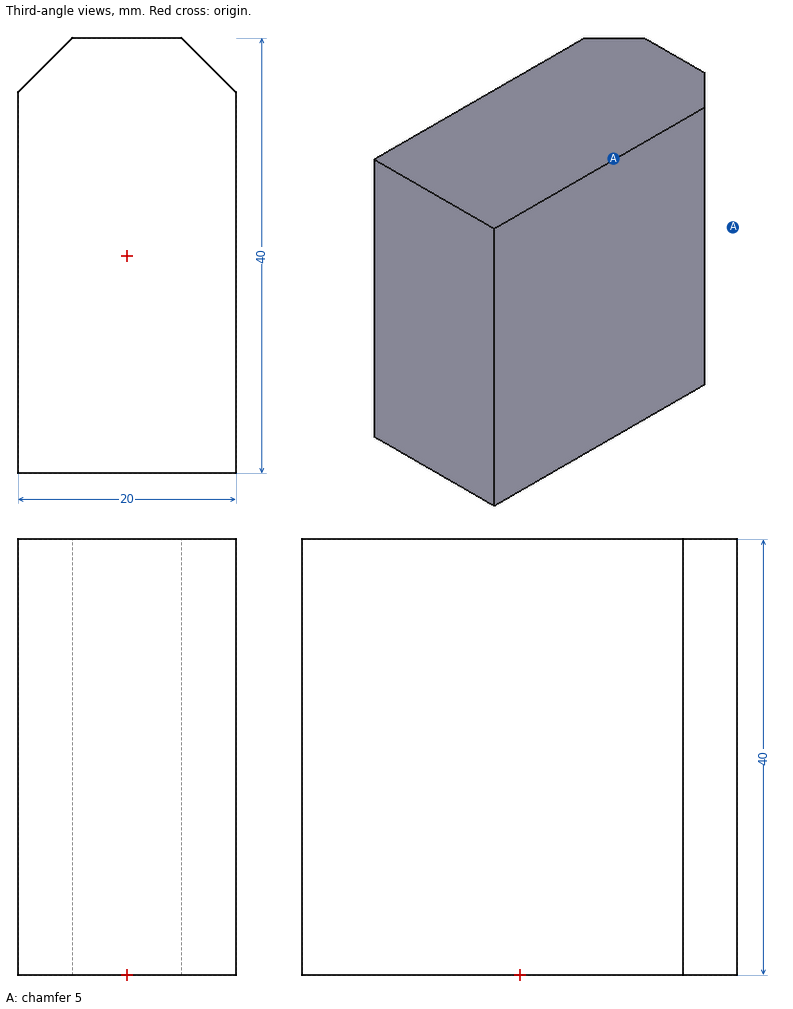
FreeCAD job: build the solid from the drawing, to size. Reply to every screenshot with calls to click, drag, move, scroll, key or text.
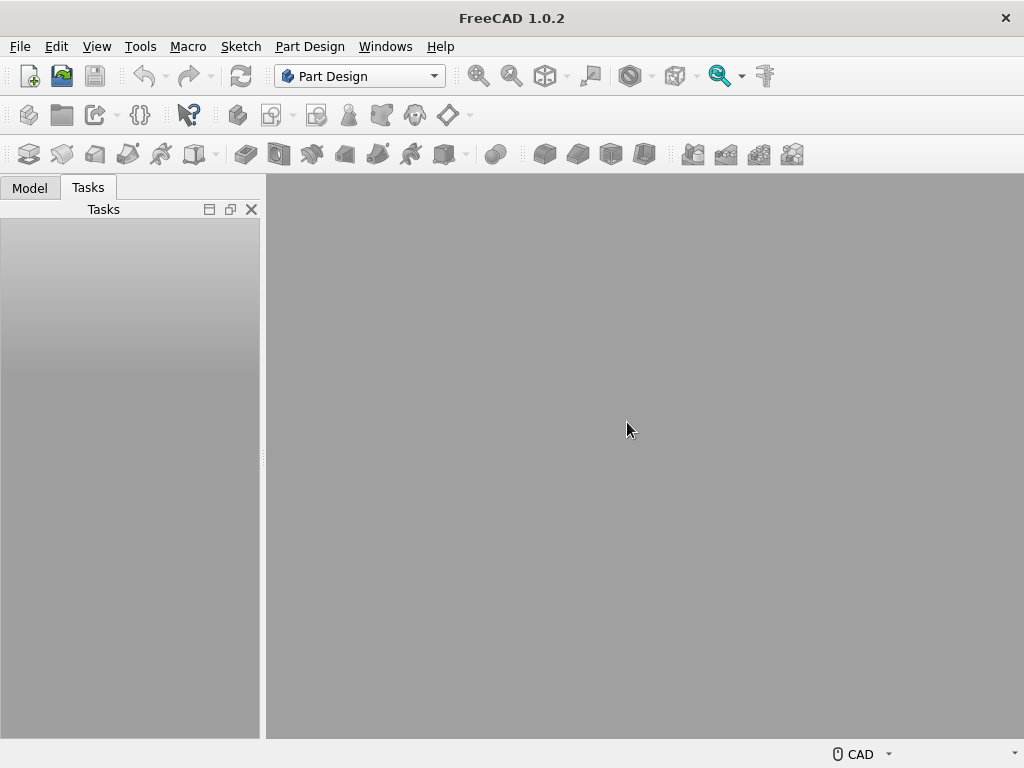
click(29, 76)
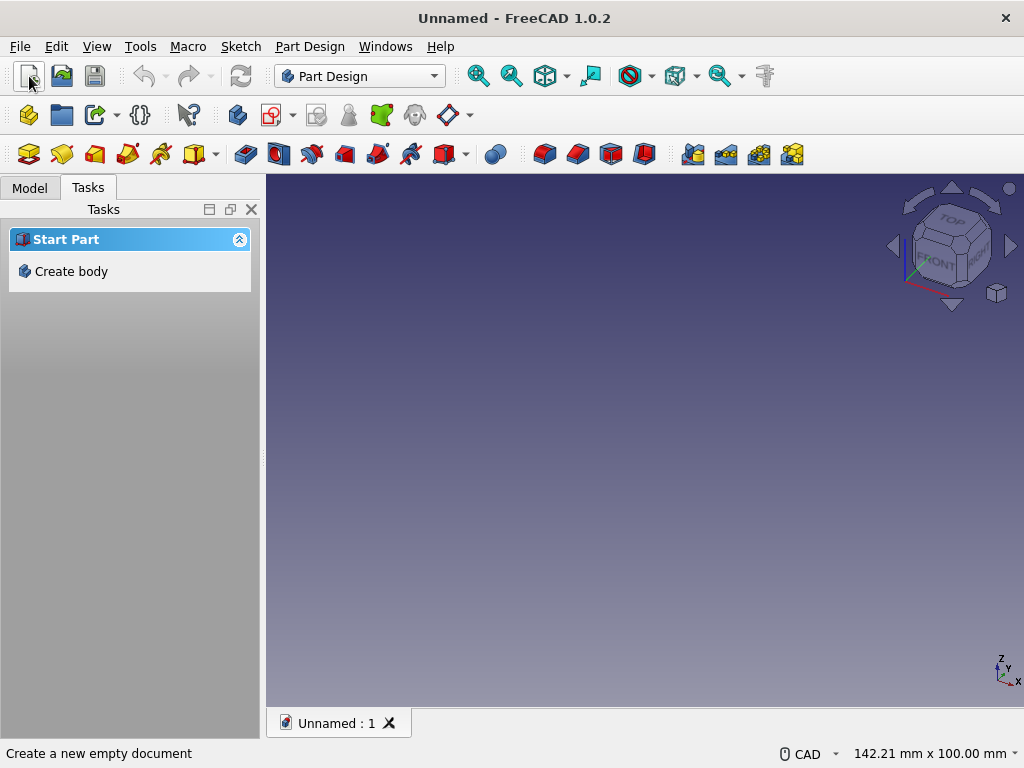
click(270, 116)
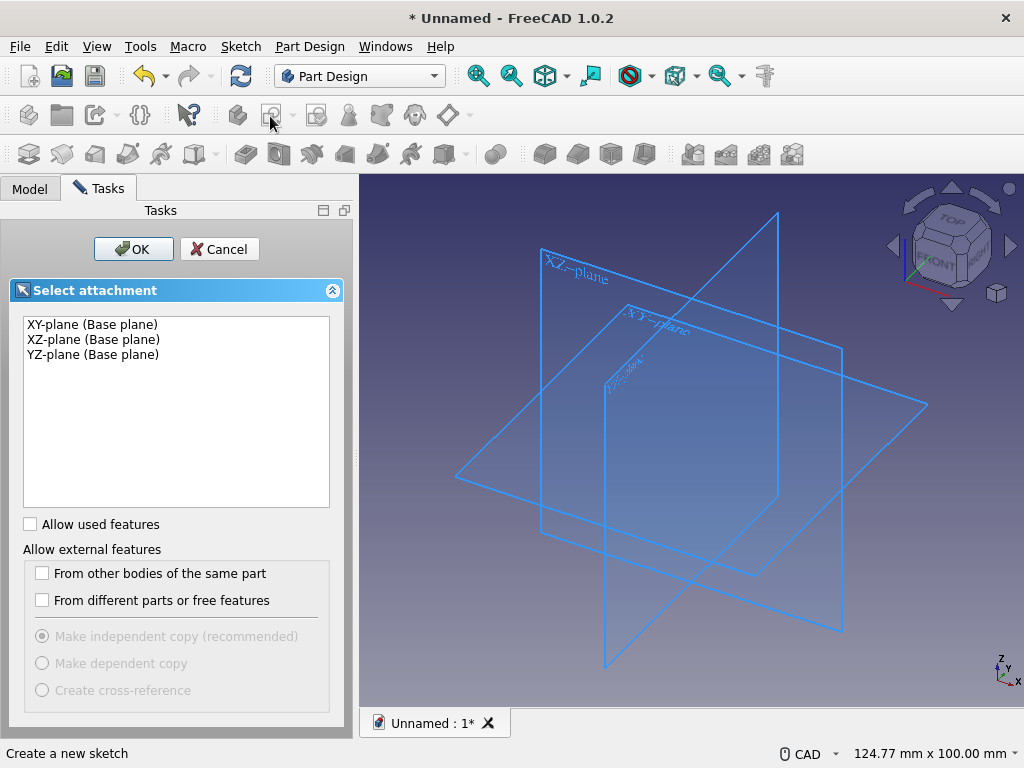
click(84, 324)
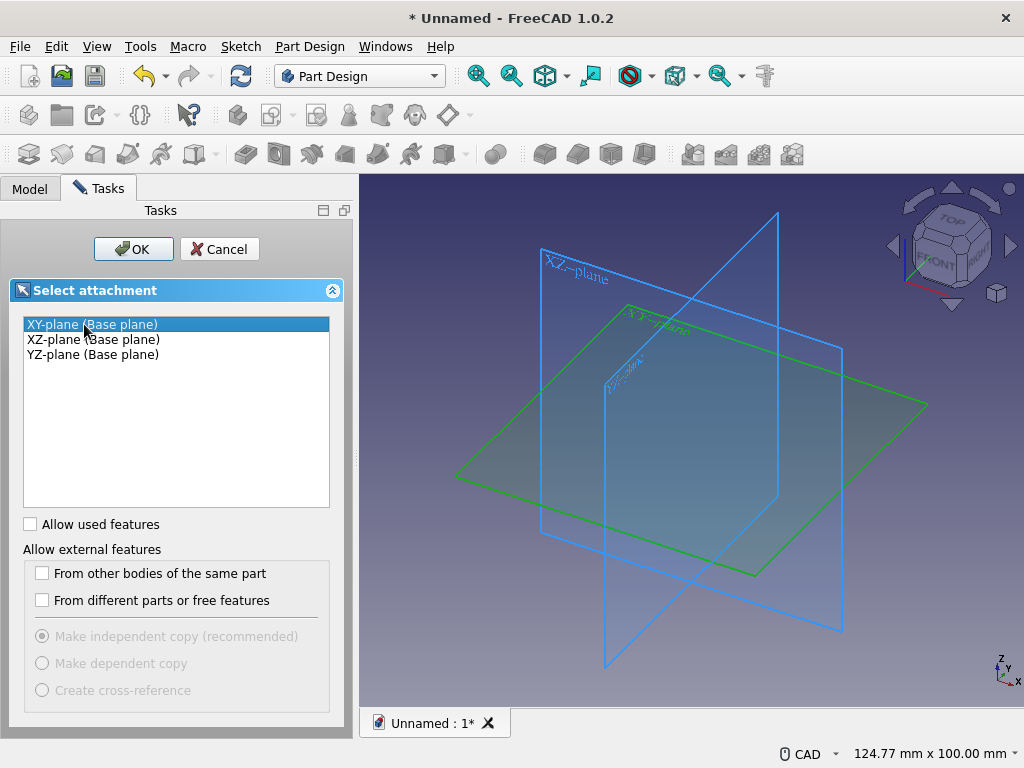
click(134, 249)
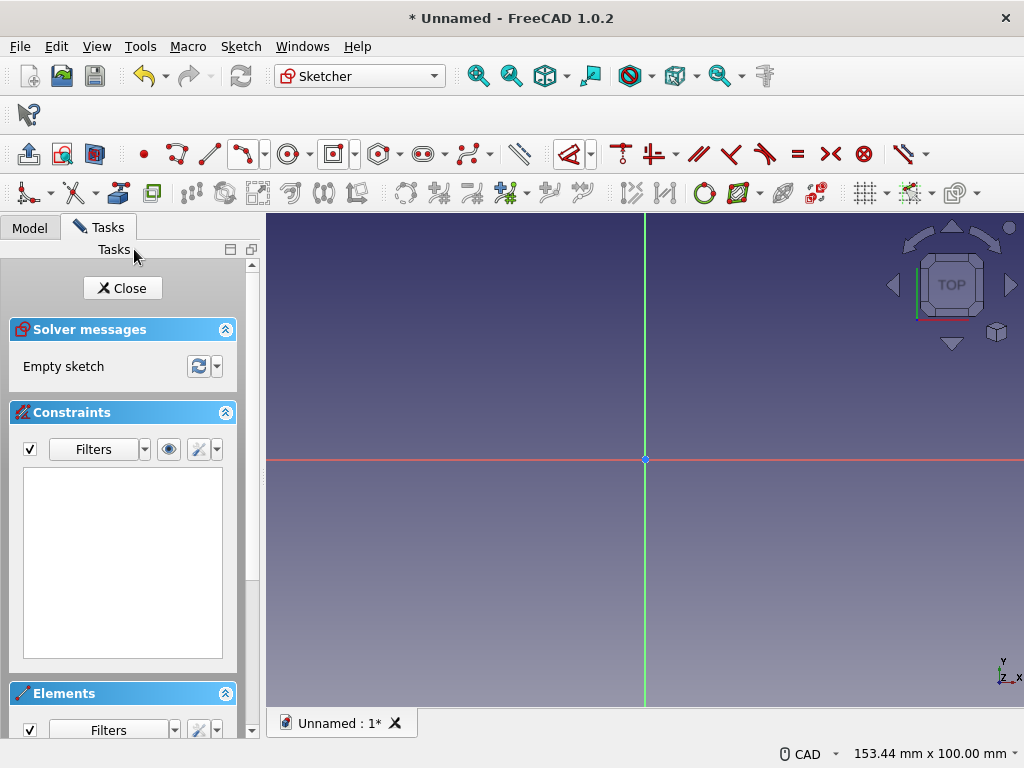
scroll(784, 460, up, 2)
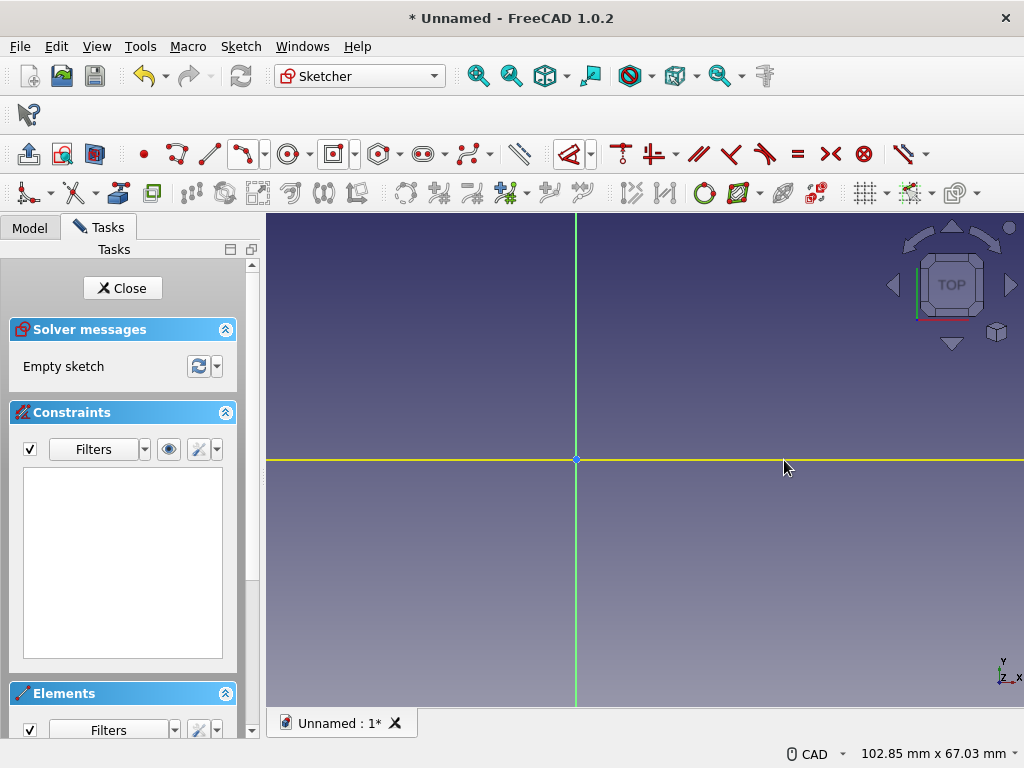
click(332, 154)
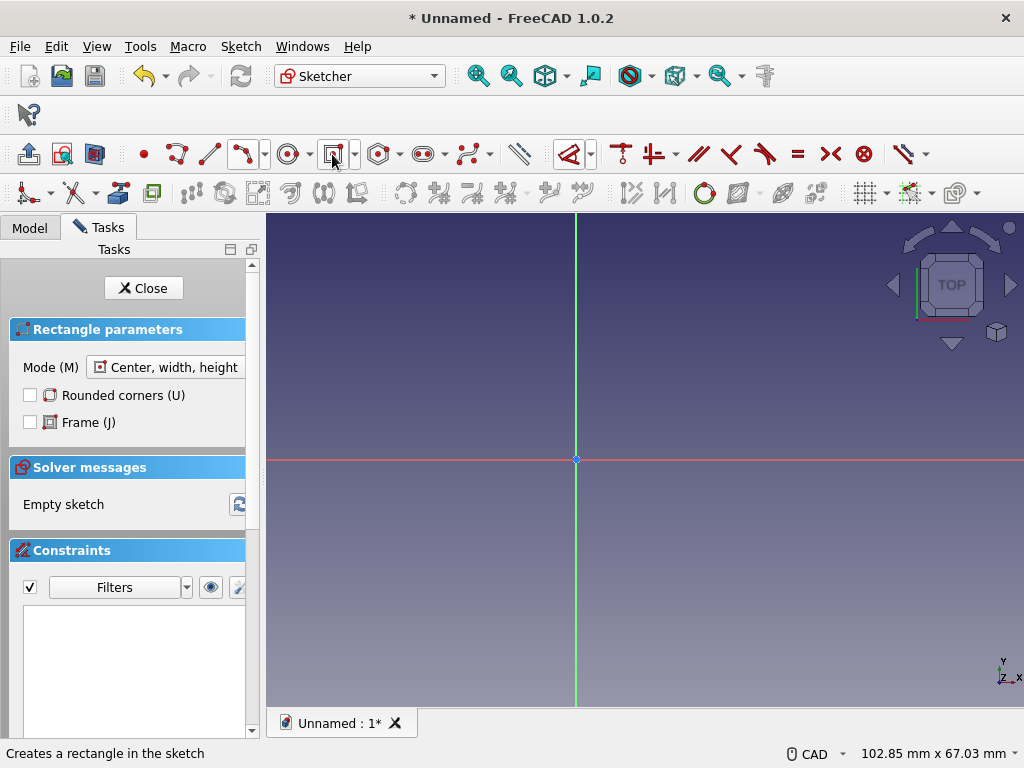
click(576, 460)
move(650, 312)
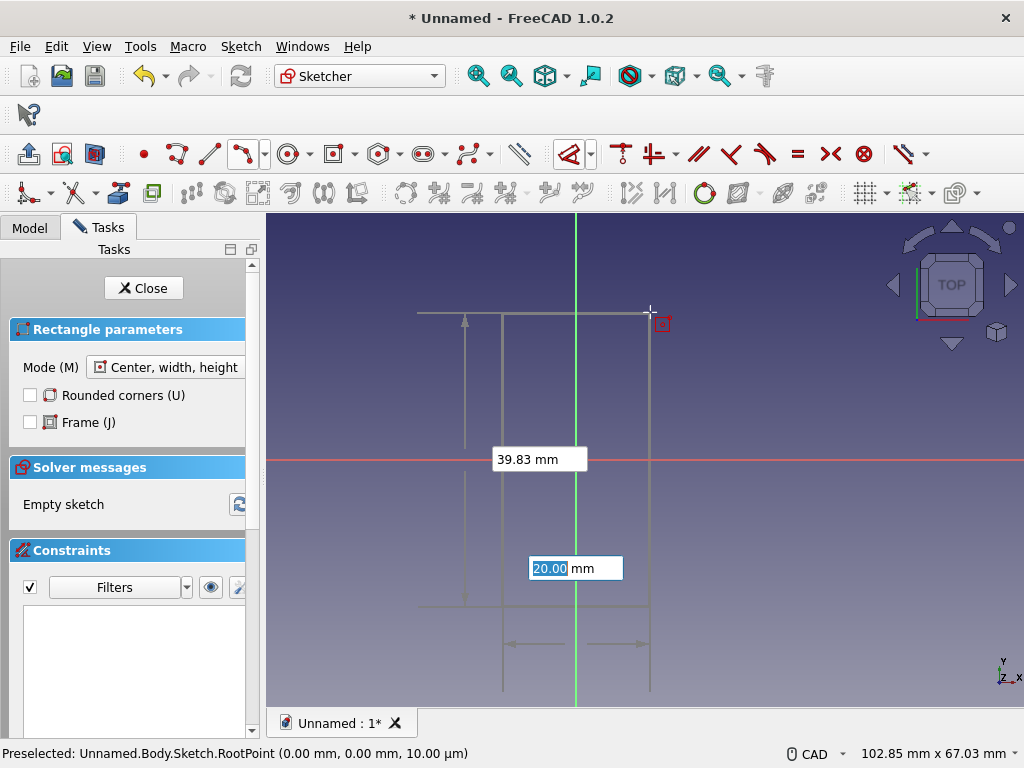
text(20)
key(Tab)
text(40)
key(Return)
key(Escape)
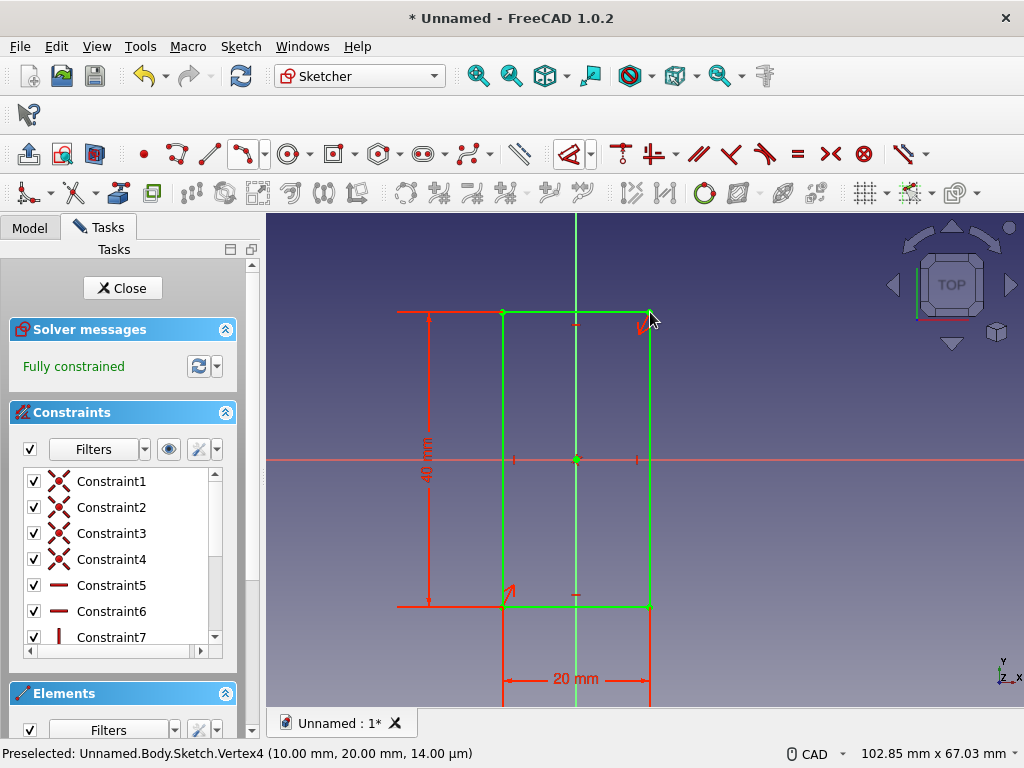
click(123, 288)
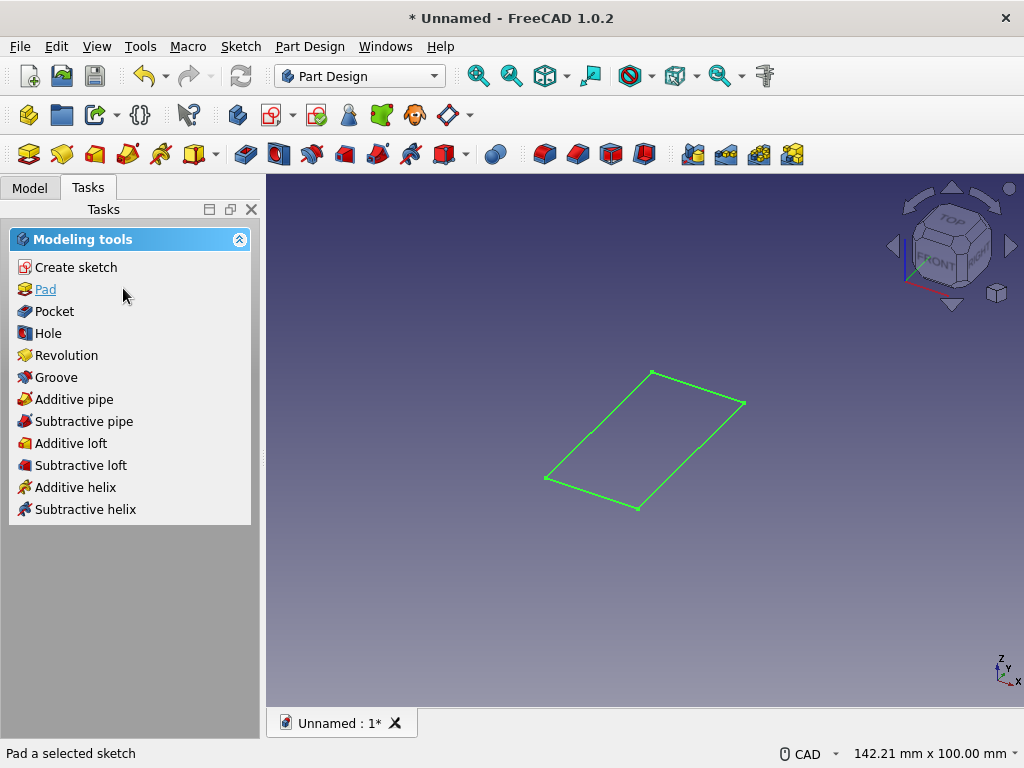
click(29, 154)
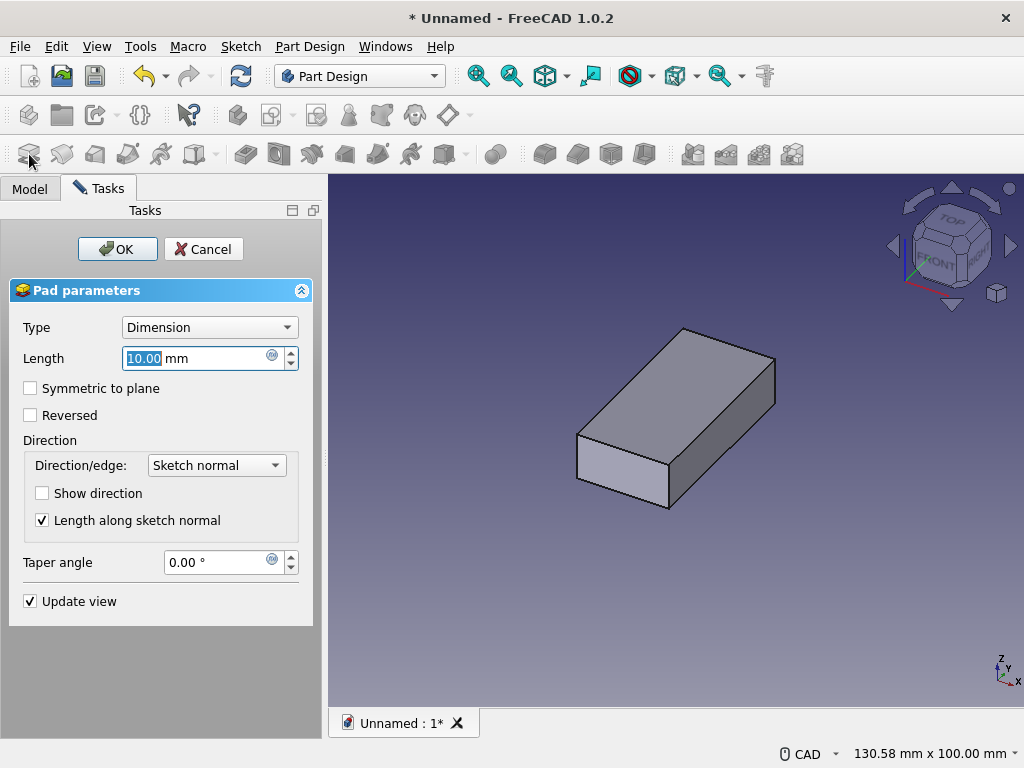
text(40)
key(Tab)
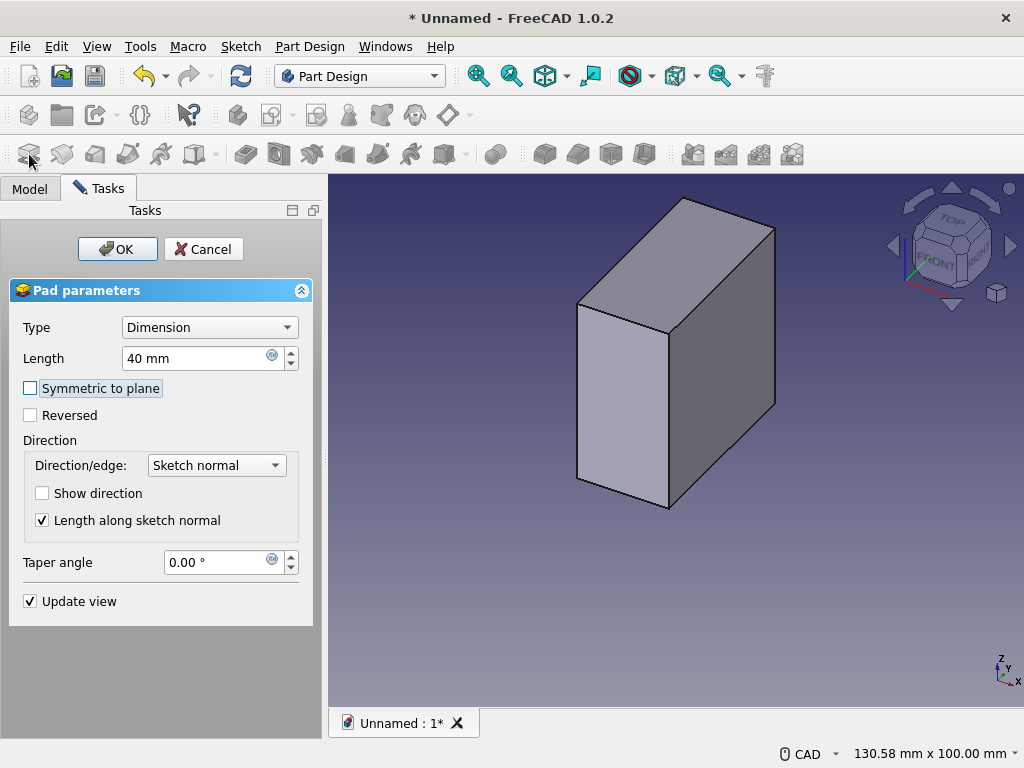
click(118, 249)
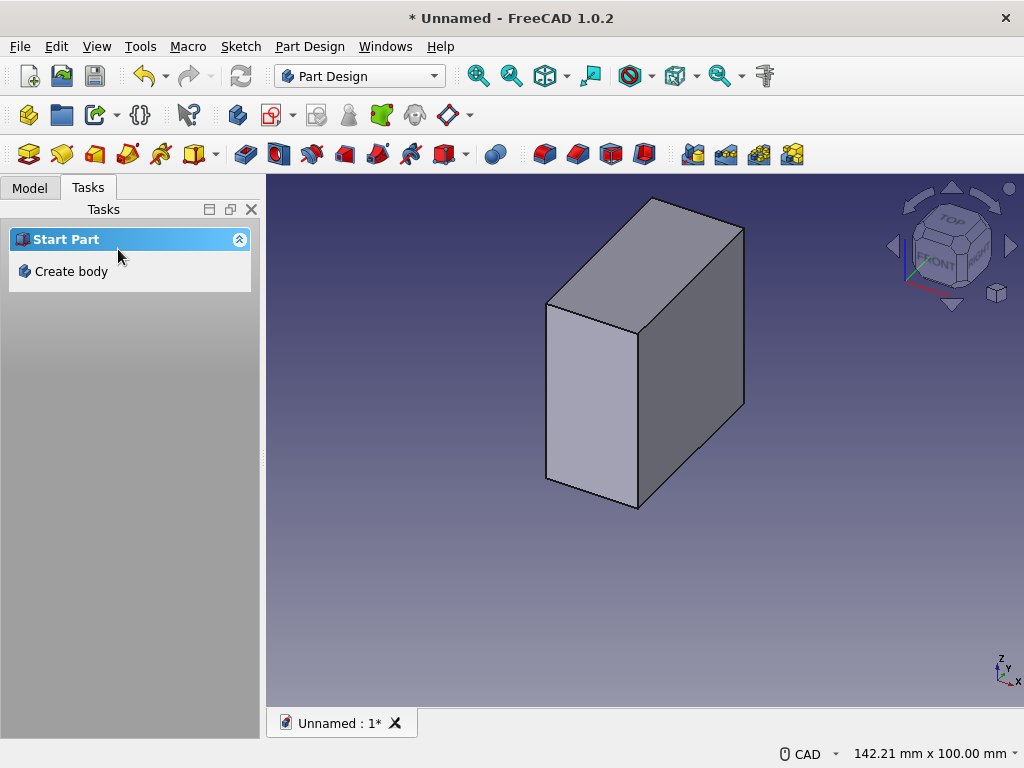
key(0)